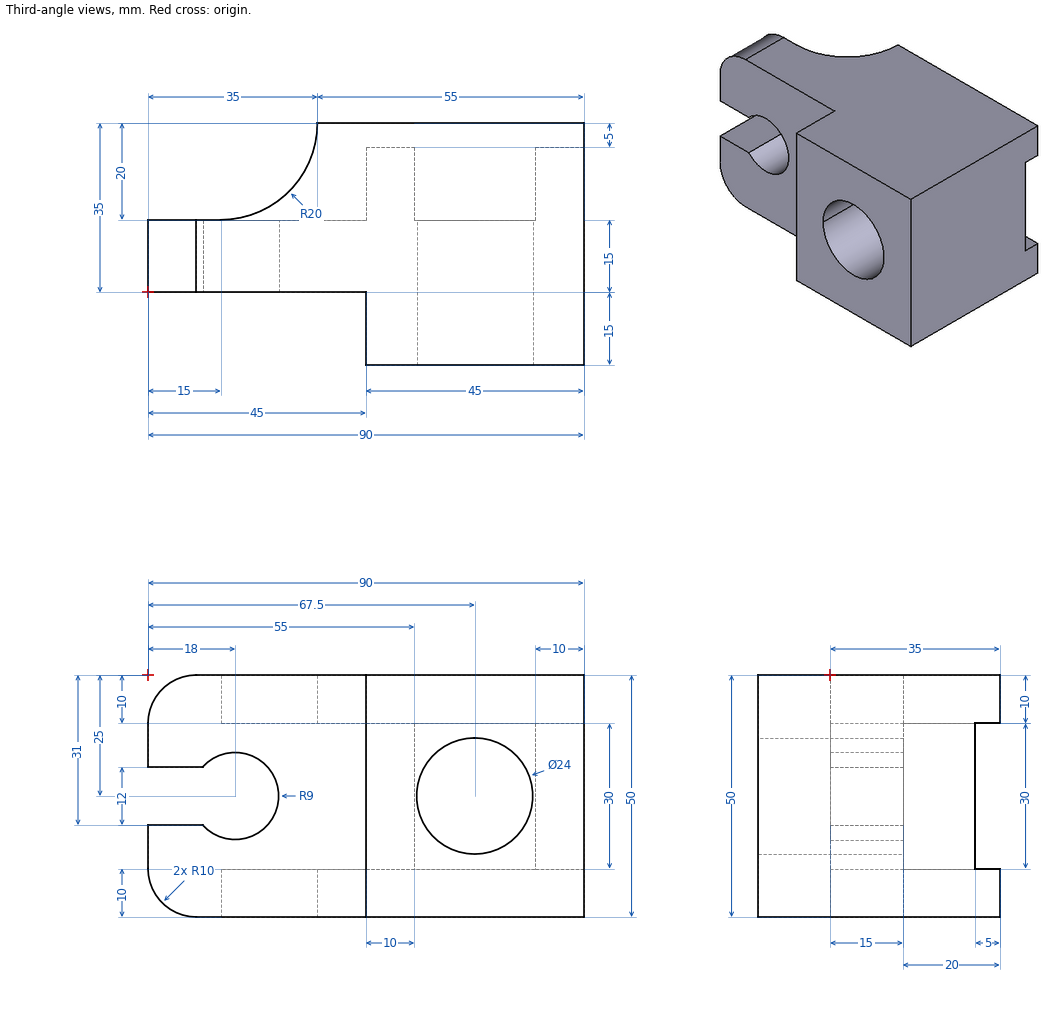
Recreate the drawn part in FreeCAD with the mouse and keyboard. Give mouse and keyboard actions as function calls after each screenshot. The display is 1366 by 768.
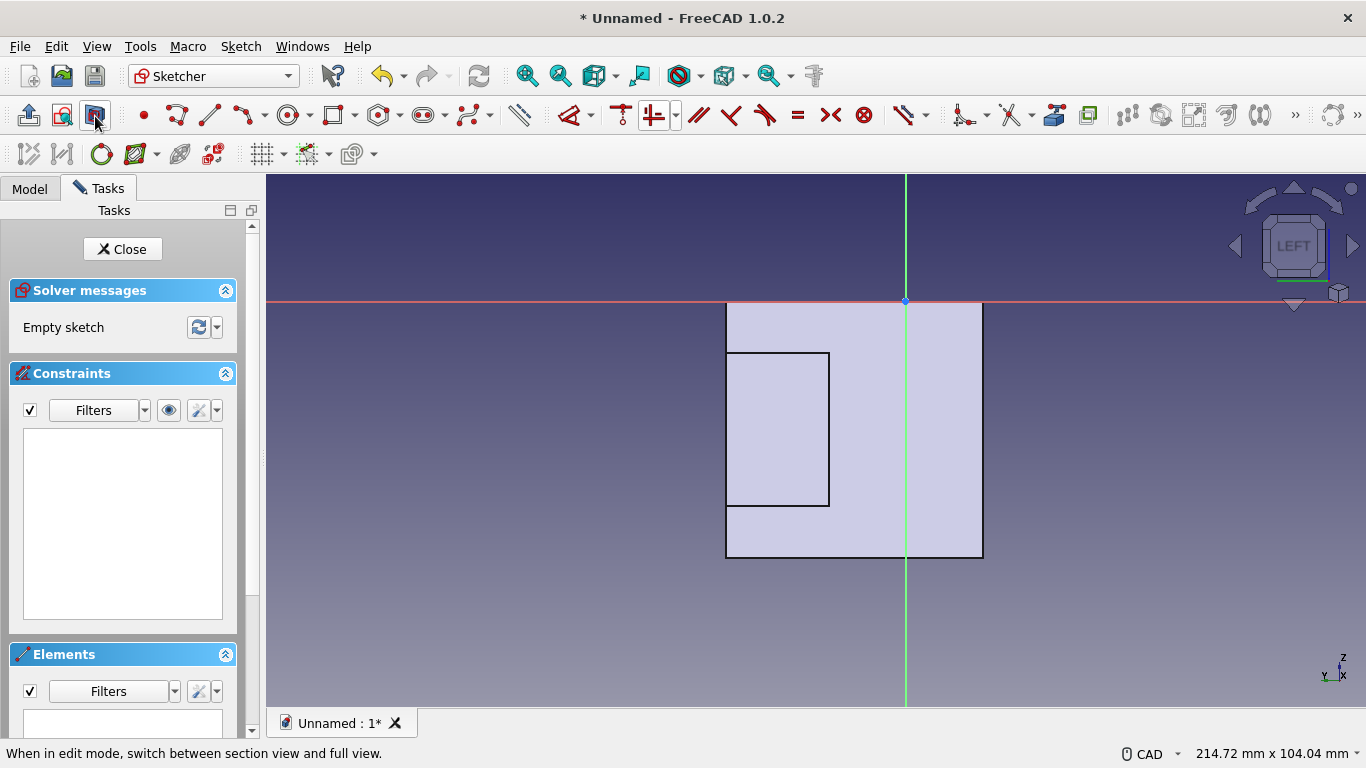
scroll(956, 330, up, 2)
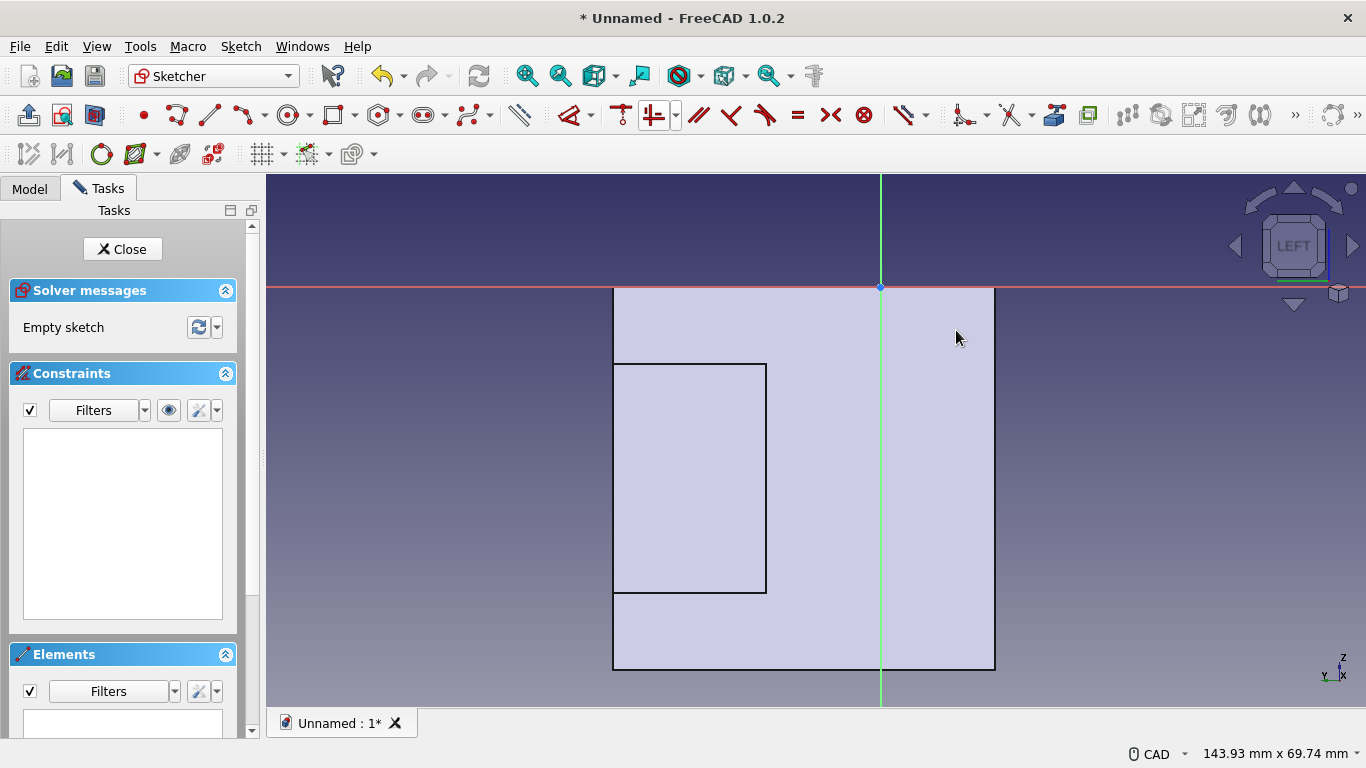
key(g)
key(r)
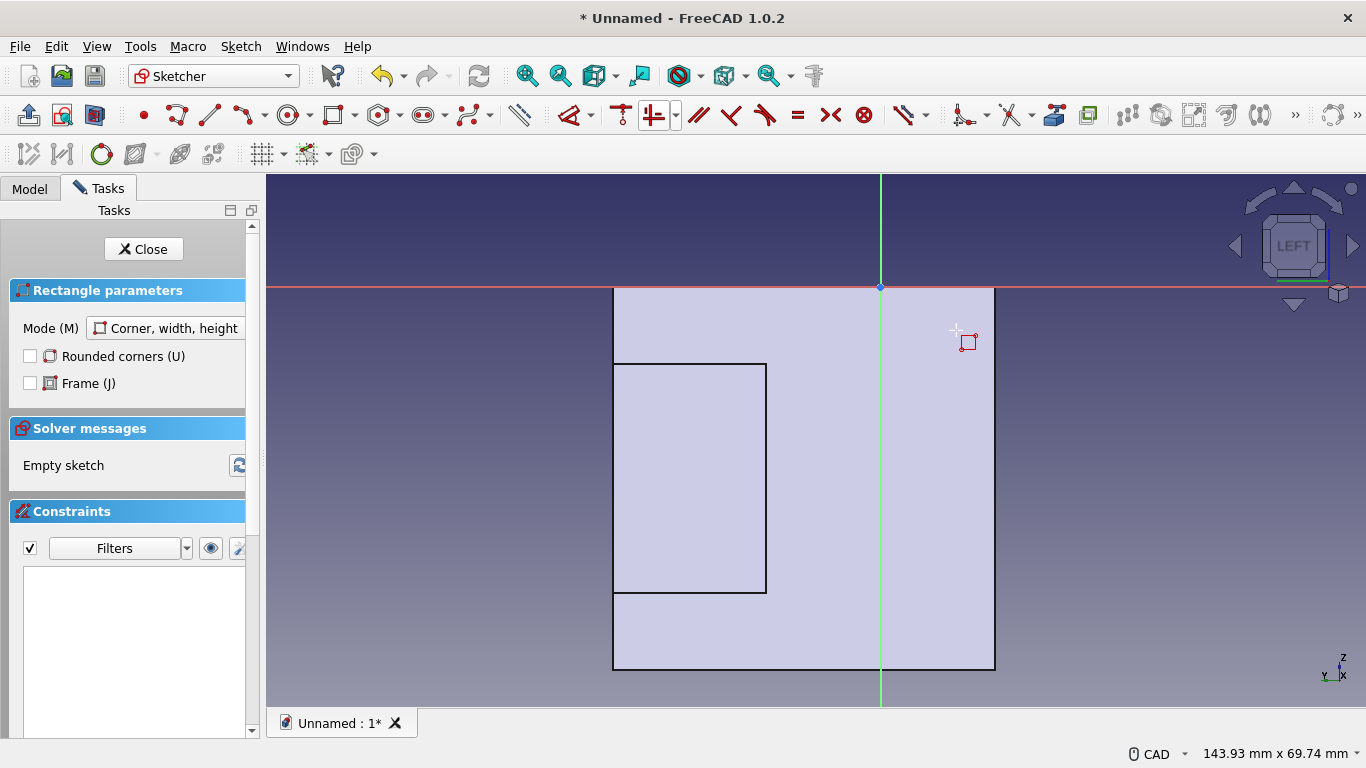
click(613, 364)
click(766, 593)
key(Escape)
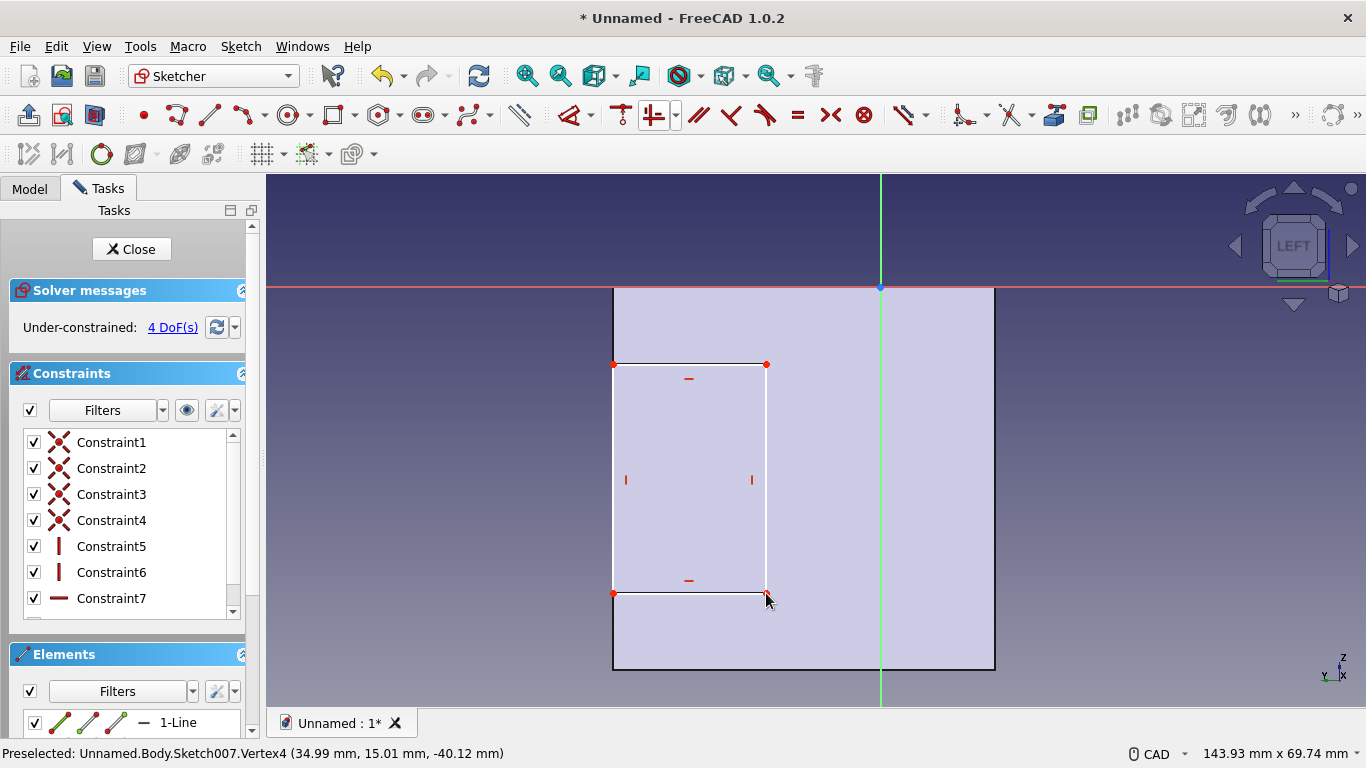
key(d)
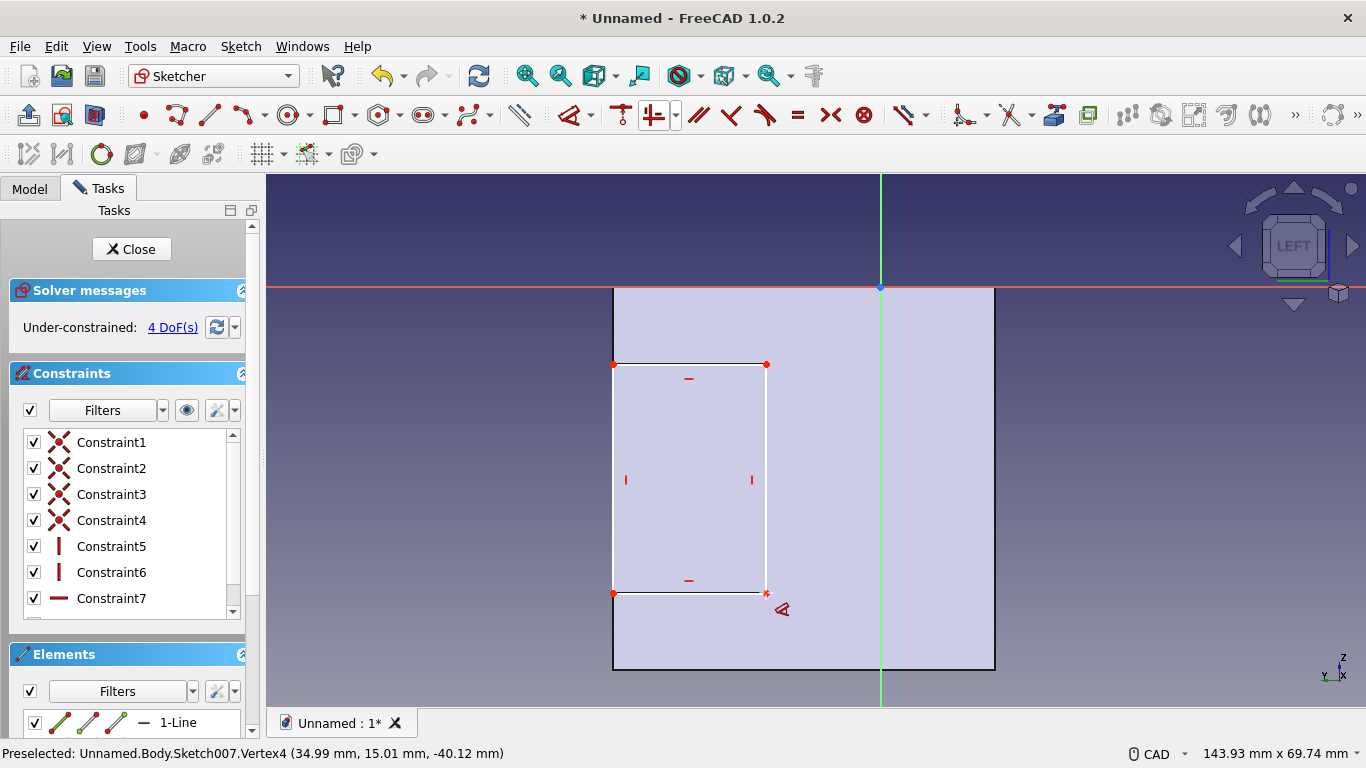
click(613, 434)
click(579, 479)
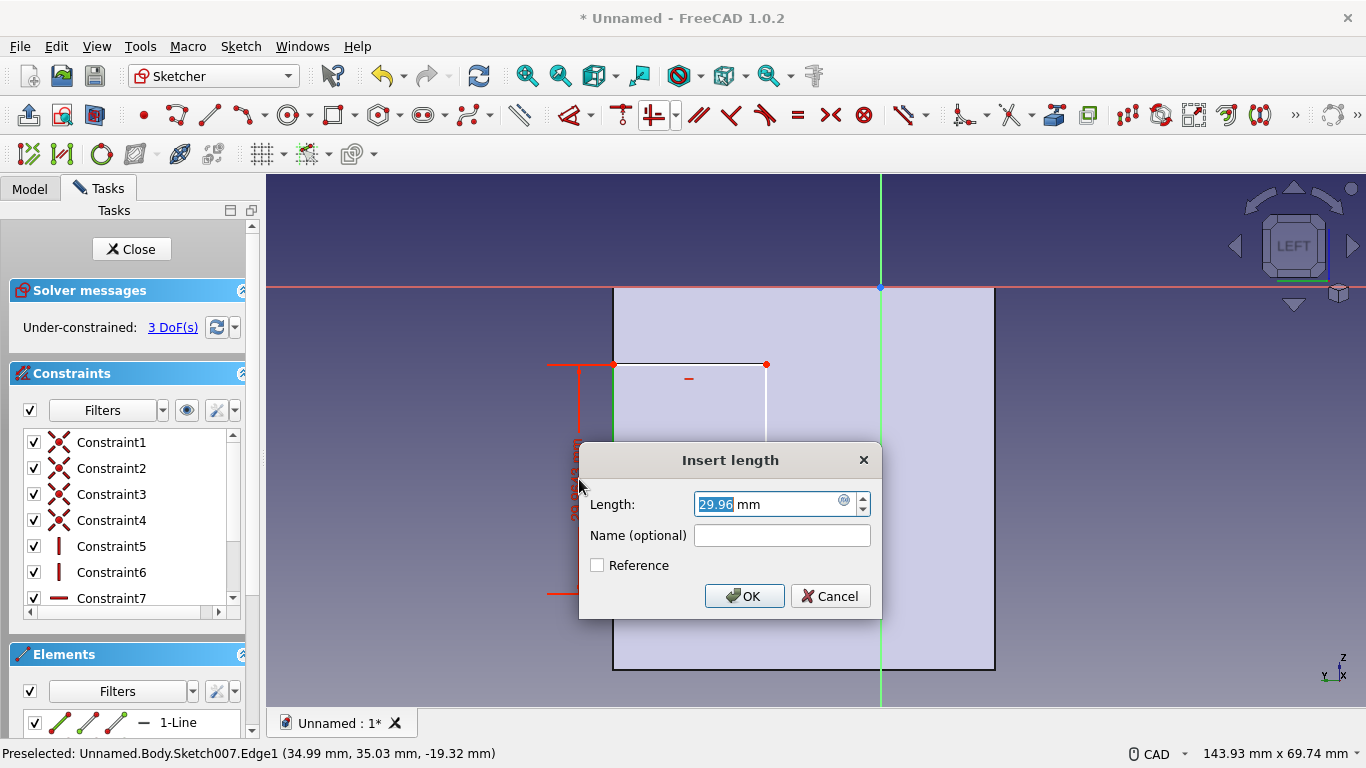
text(30)
key(Return)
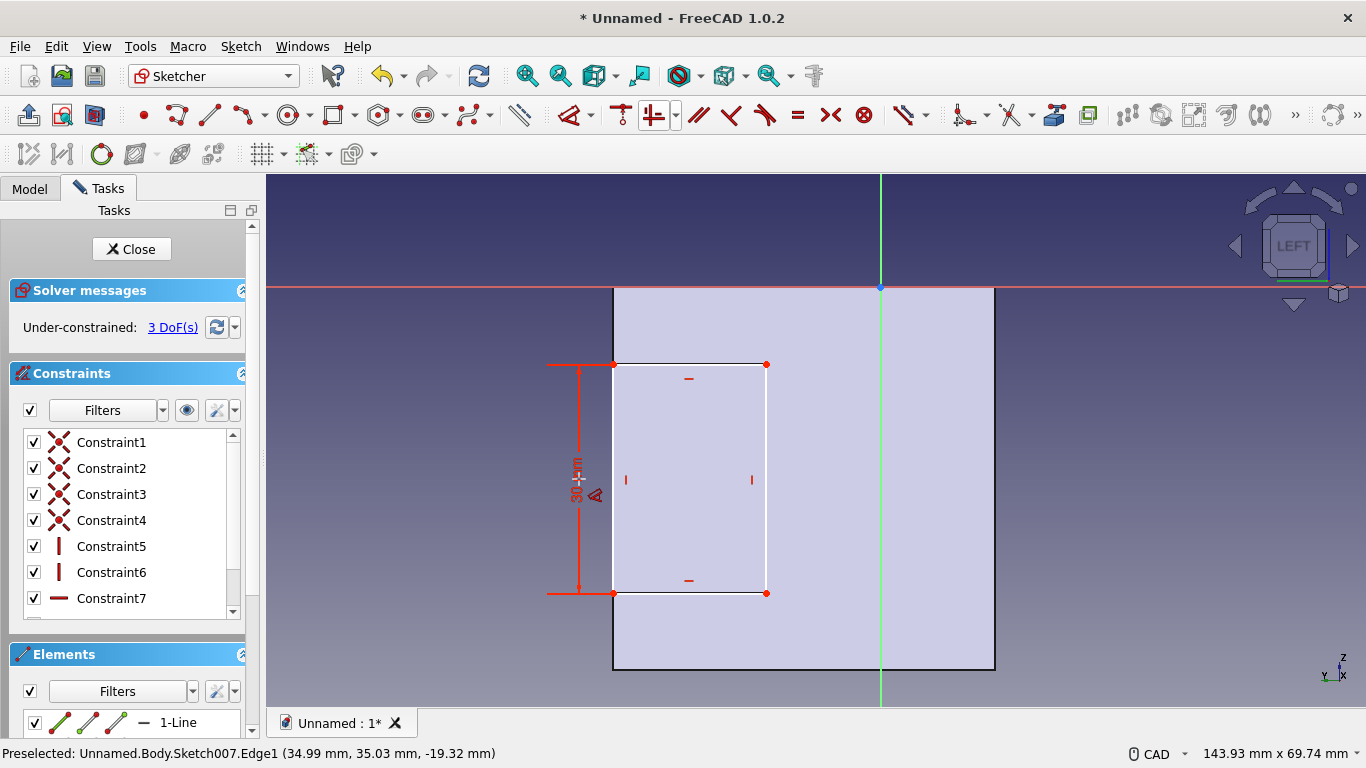
click(659, 594)
click(690, 628)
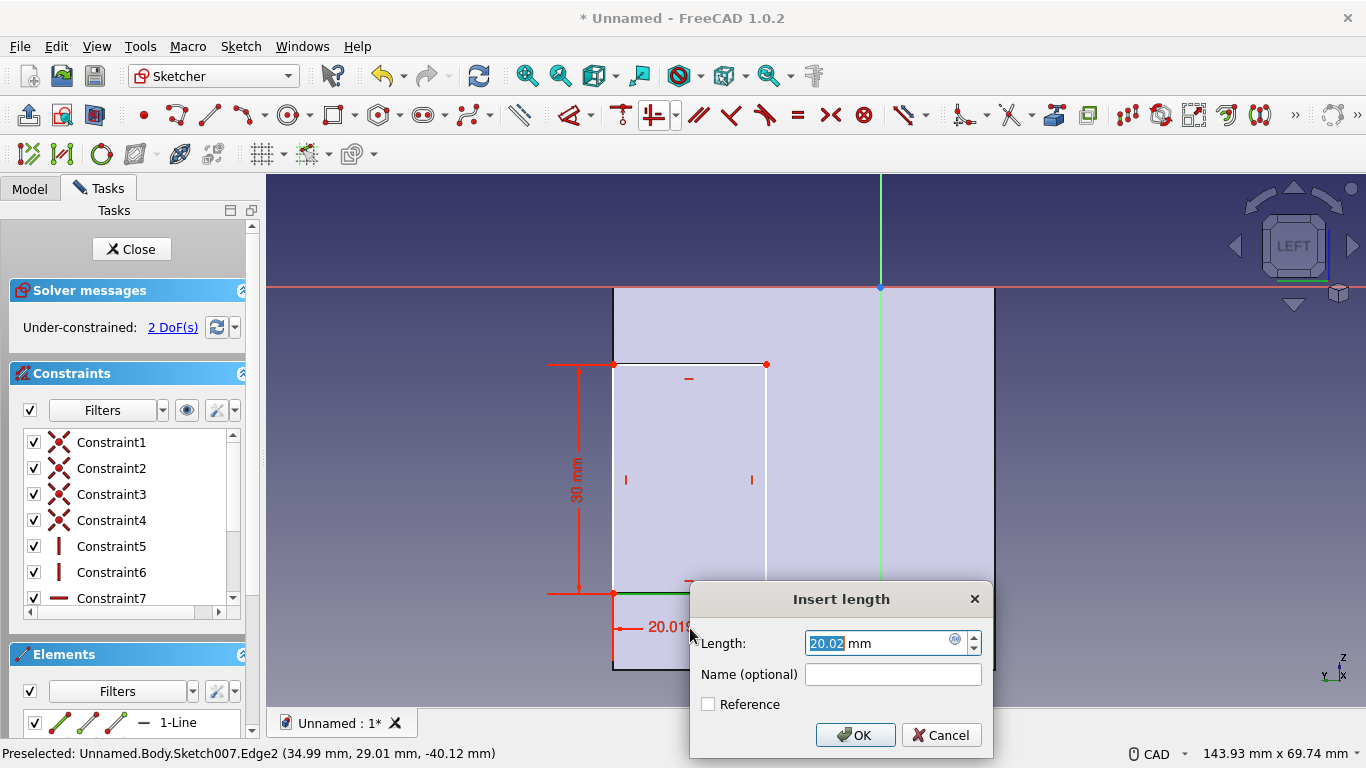
text(20)
key(Return)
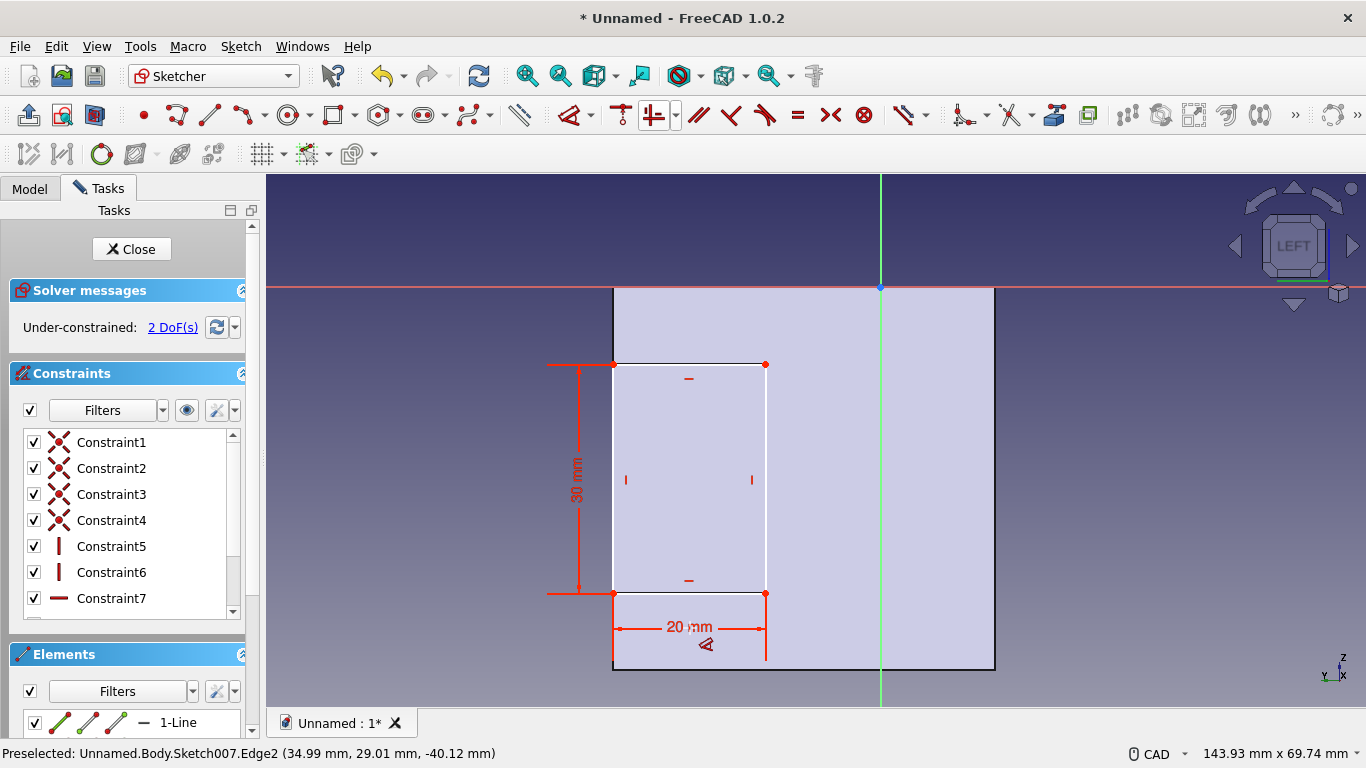
click(613, 365)
click(747, 253)